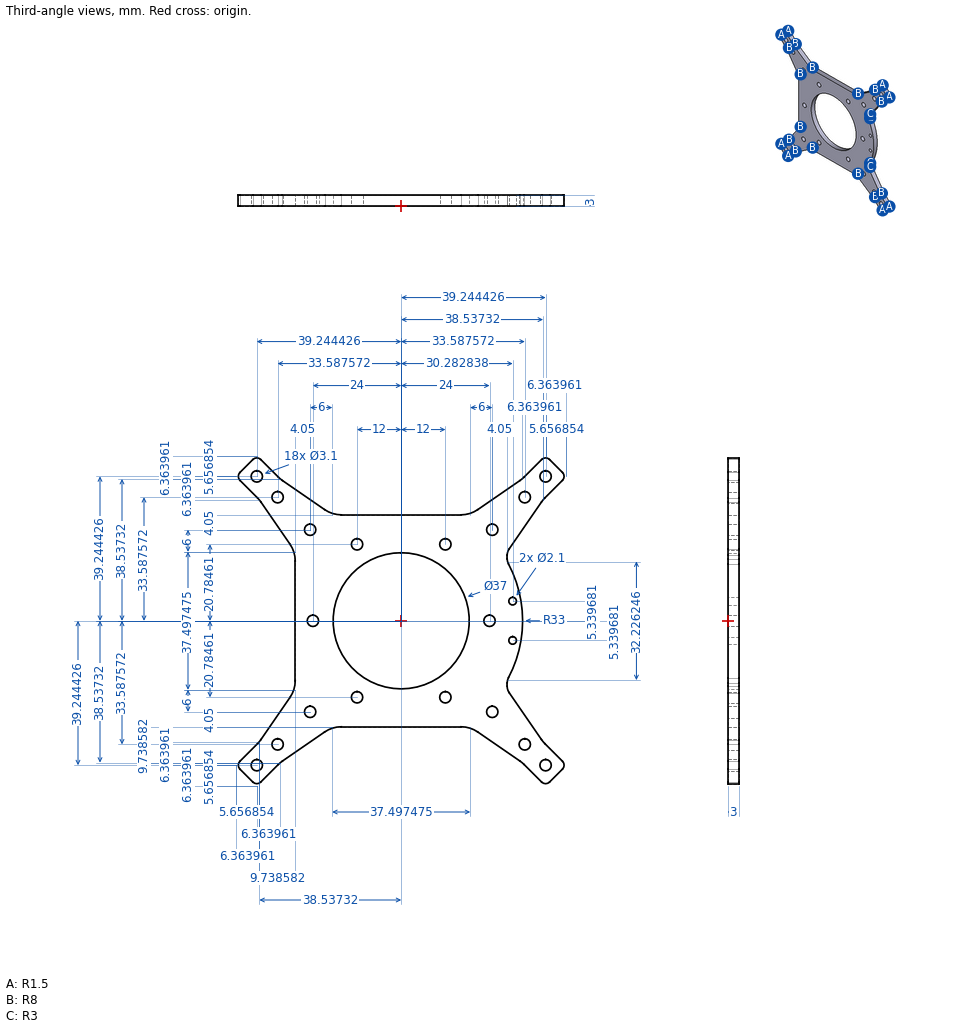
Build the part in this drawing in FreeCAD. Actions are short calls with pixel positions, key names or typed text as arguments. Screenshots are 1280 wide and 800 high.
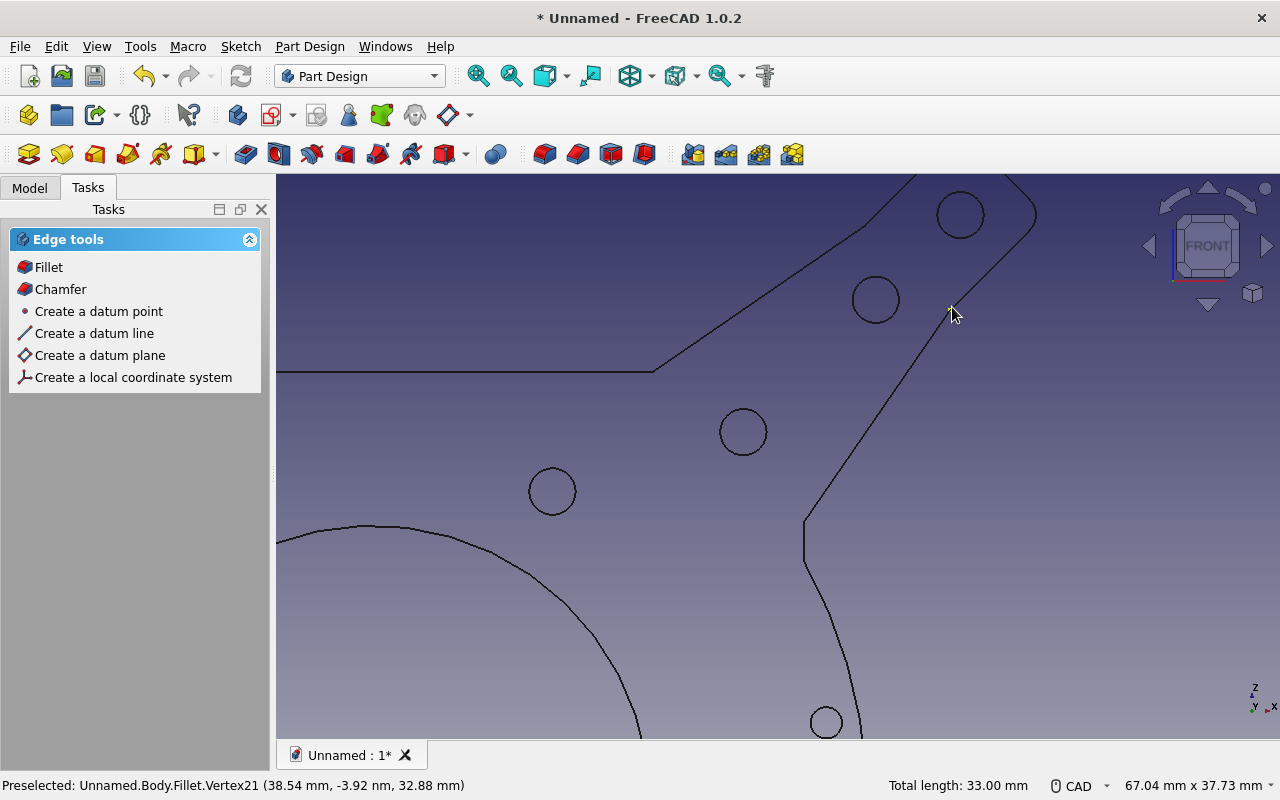
key(v)
key(f)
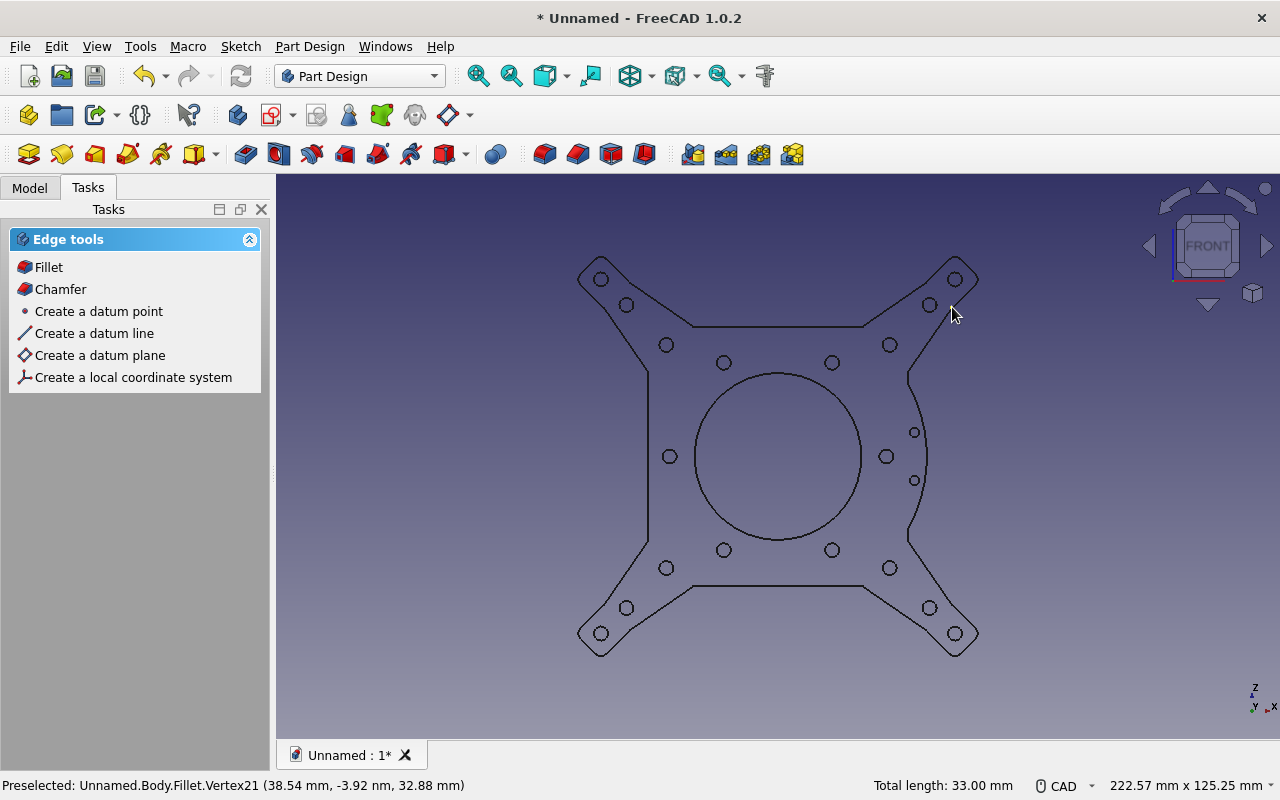
key(3)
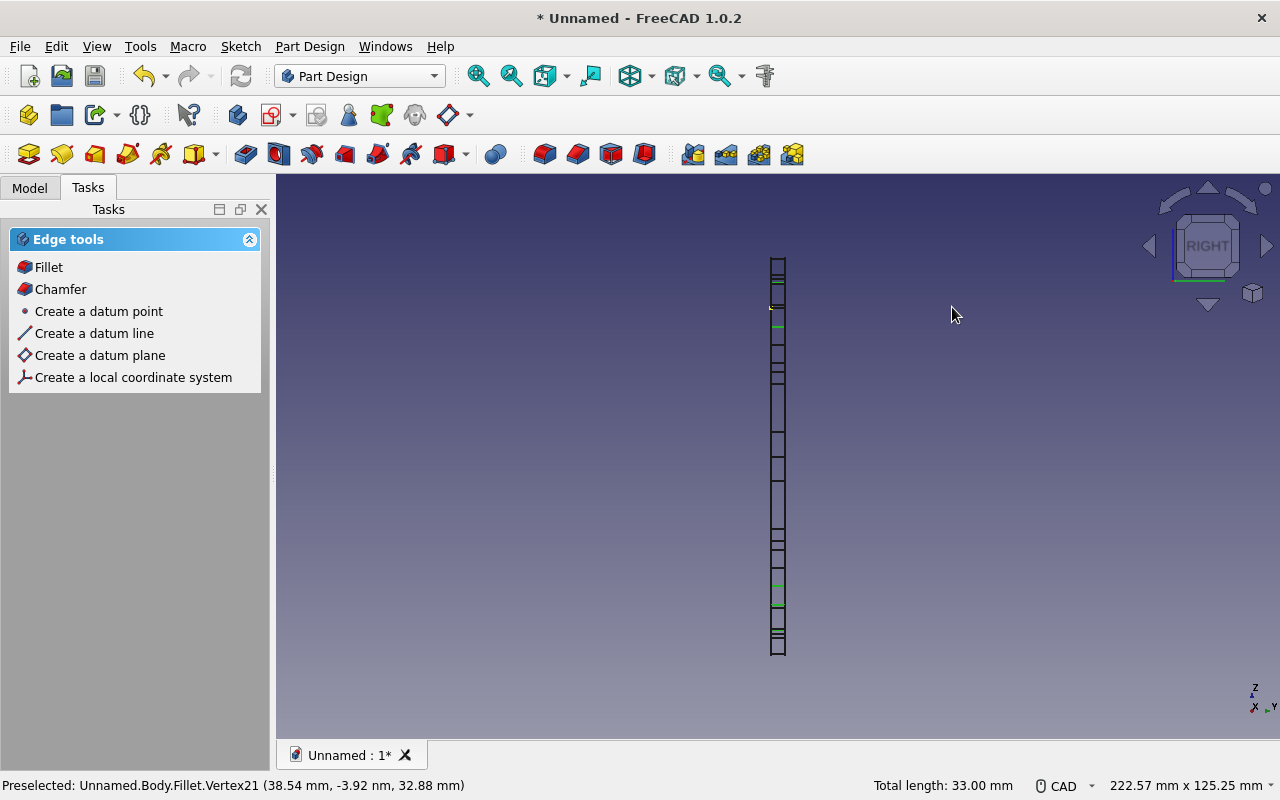
click(778, 307, ctrl)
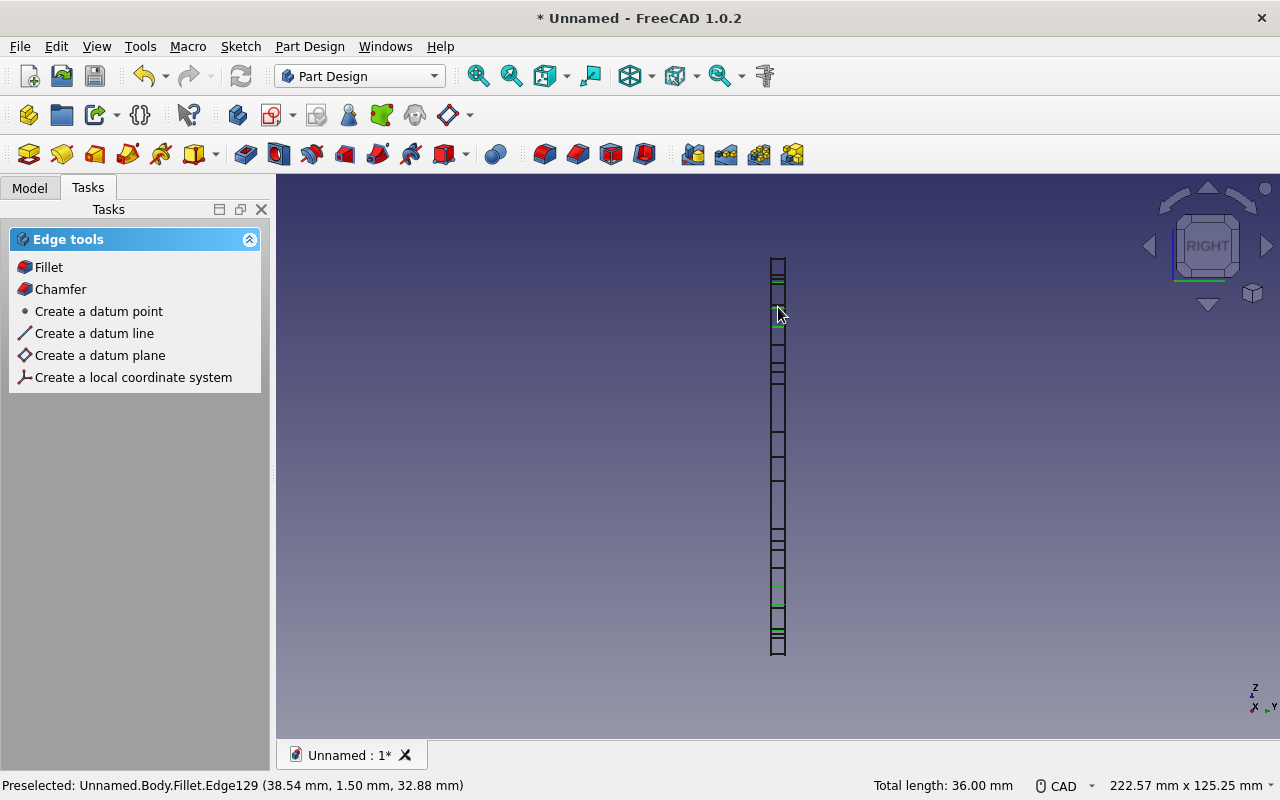
scroll(778, 604, up, 6)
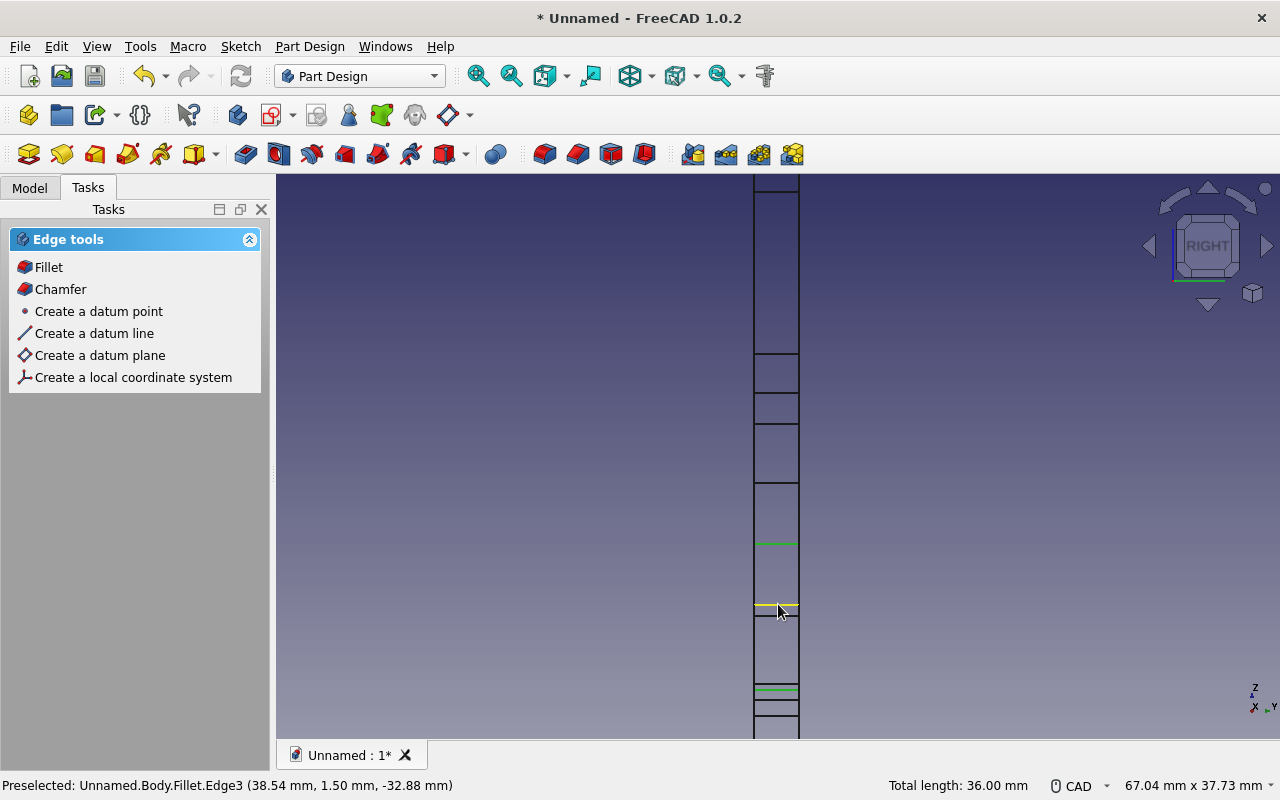
click(479, 76)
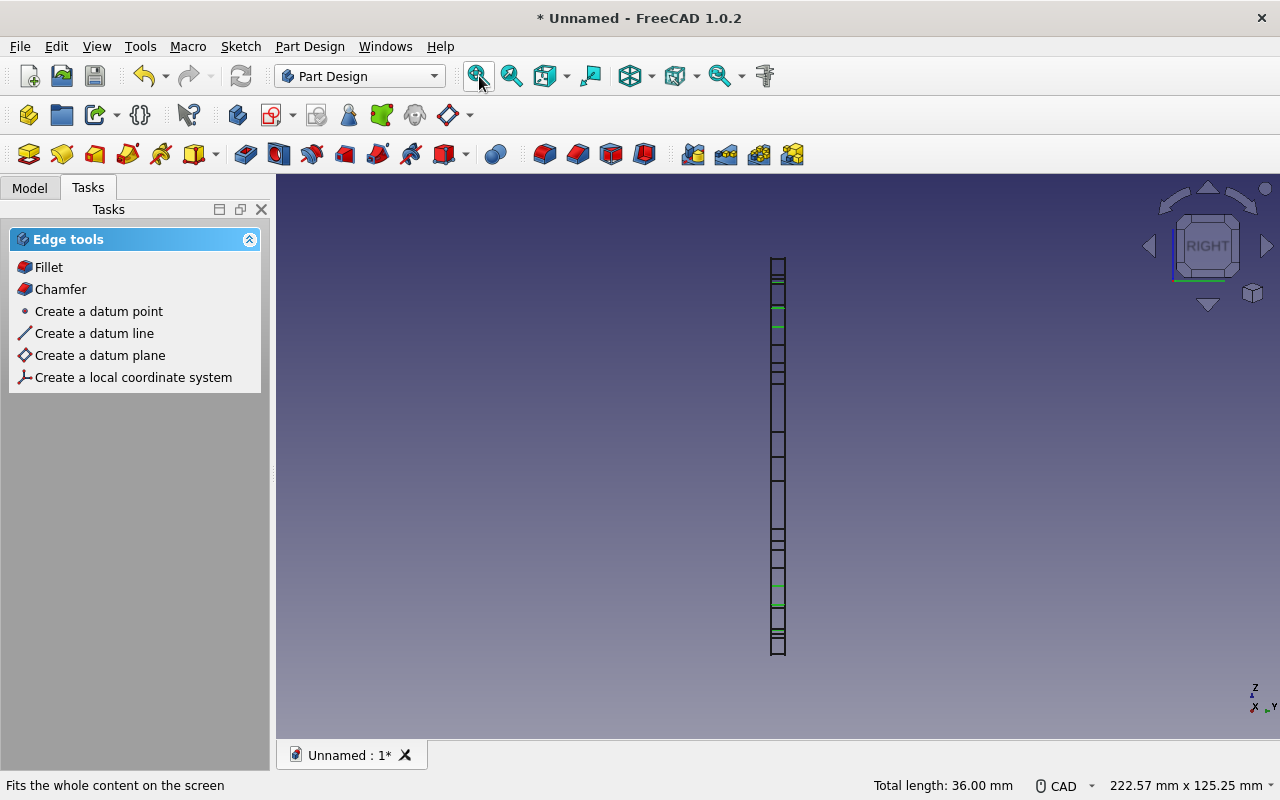
key(5)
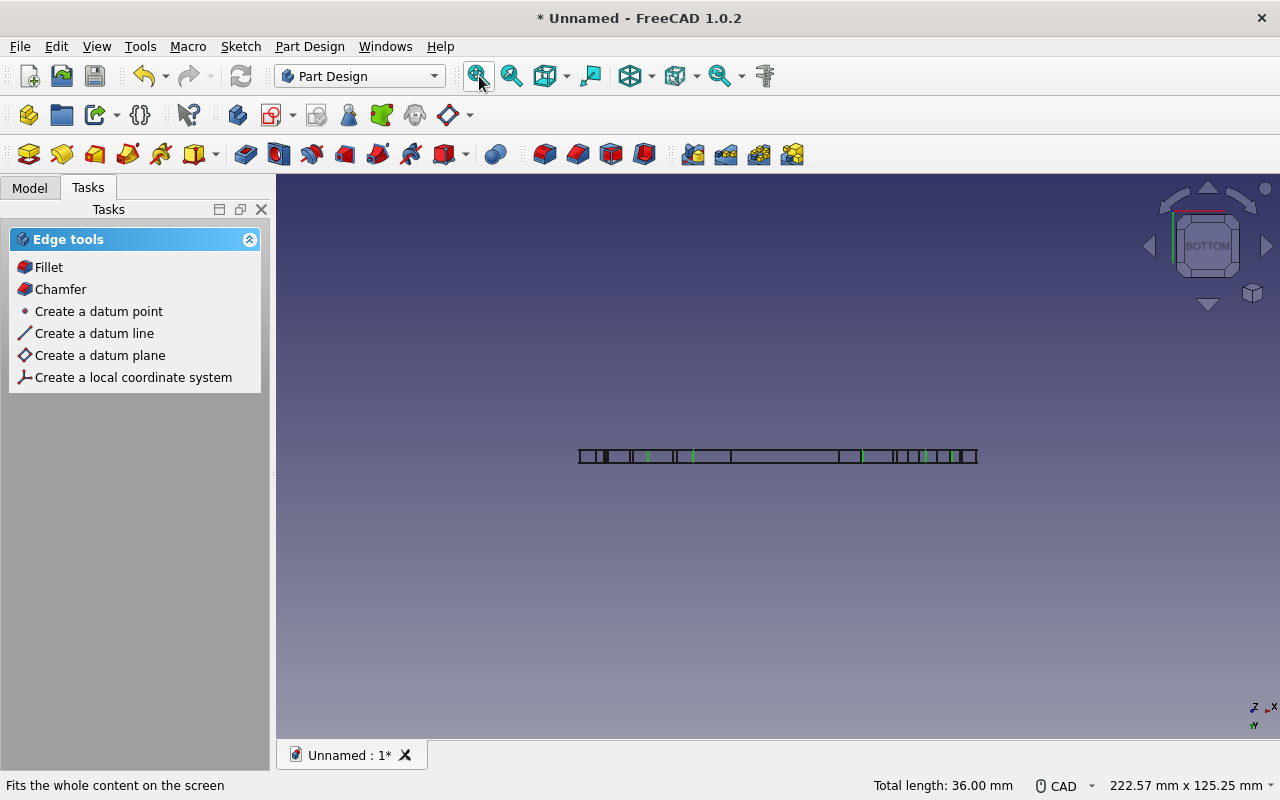
click(479, 76)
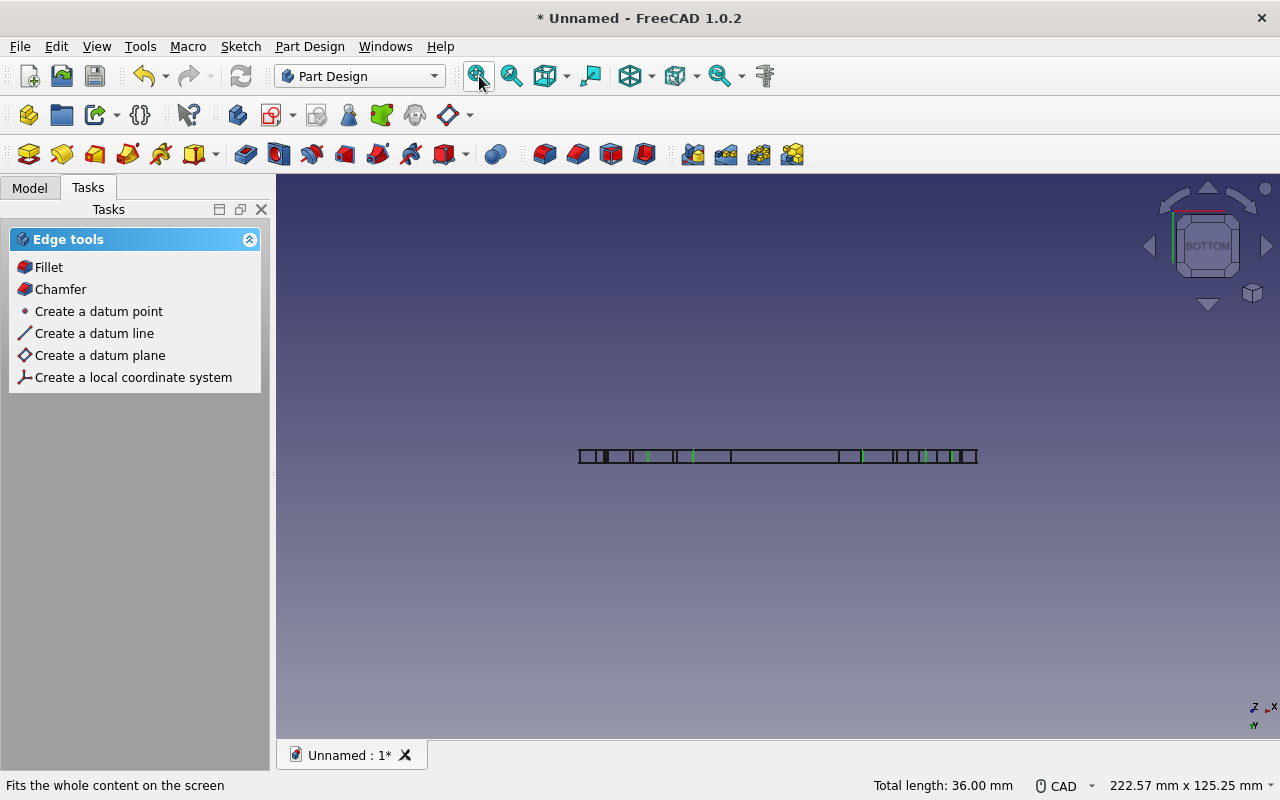
click(630, 455, ctrl)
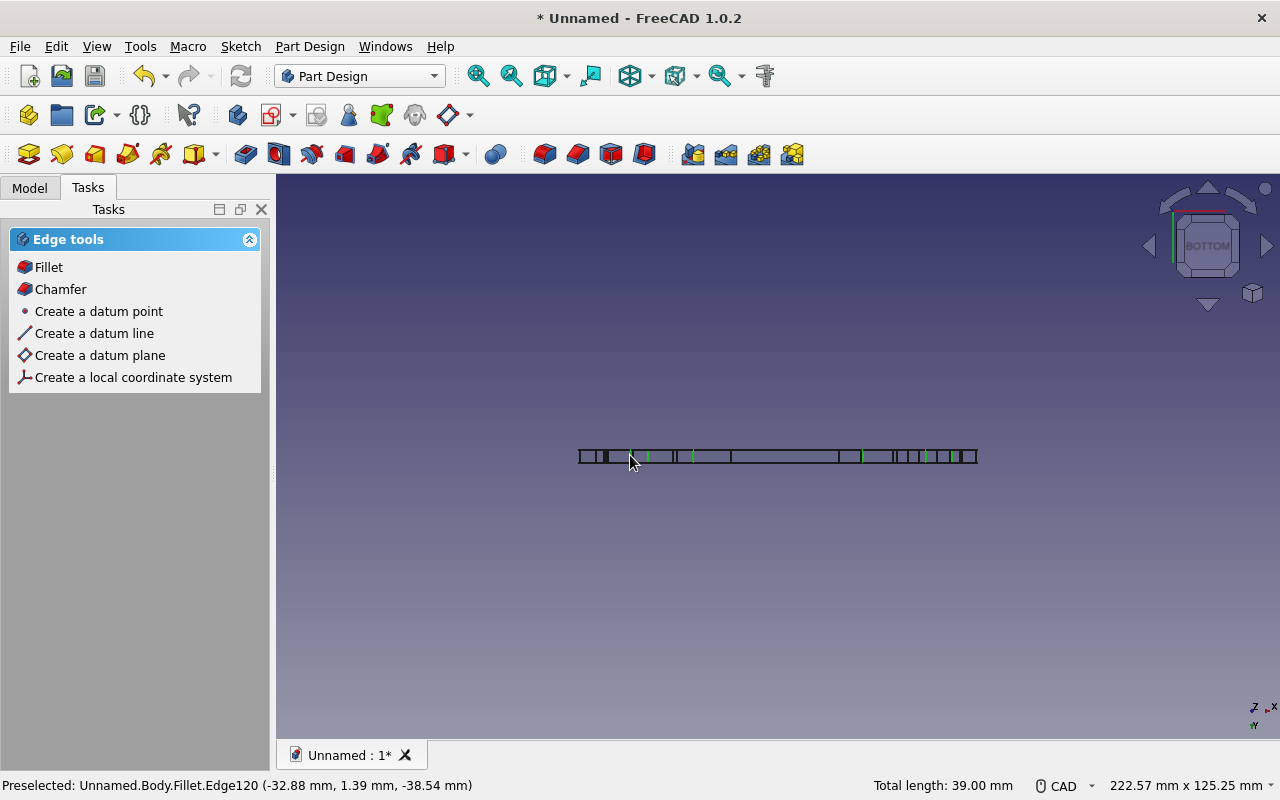
scroll(604, 455, up, 6)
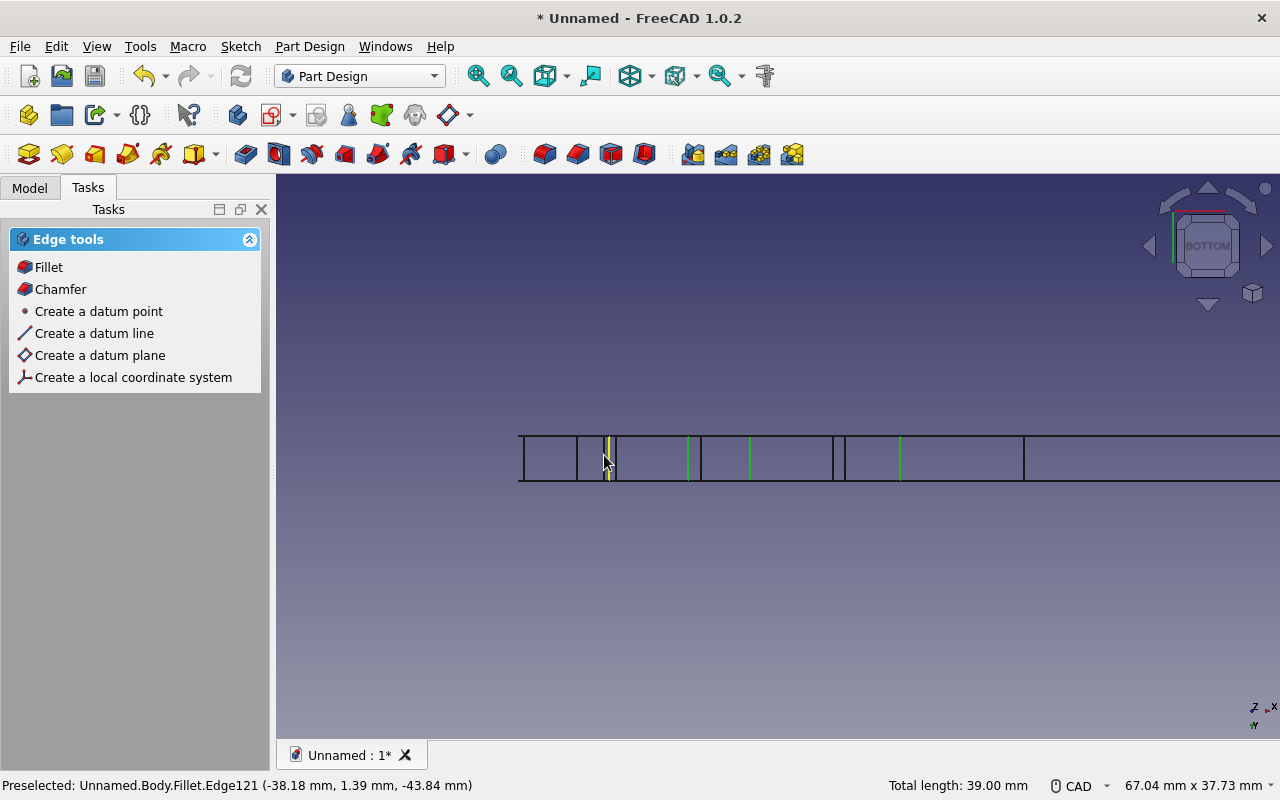
click(479, 76)